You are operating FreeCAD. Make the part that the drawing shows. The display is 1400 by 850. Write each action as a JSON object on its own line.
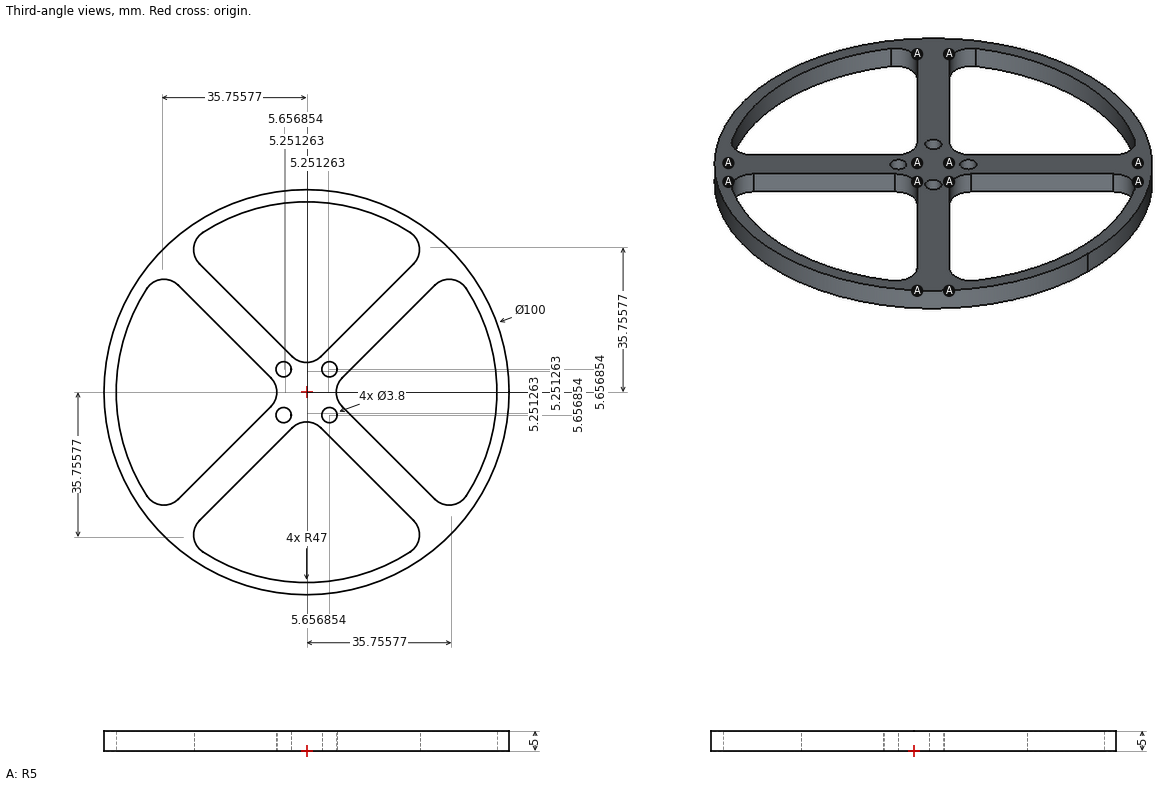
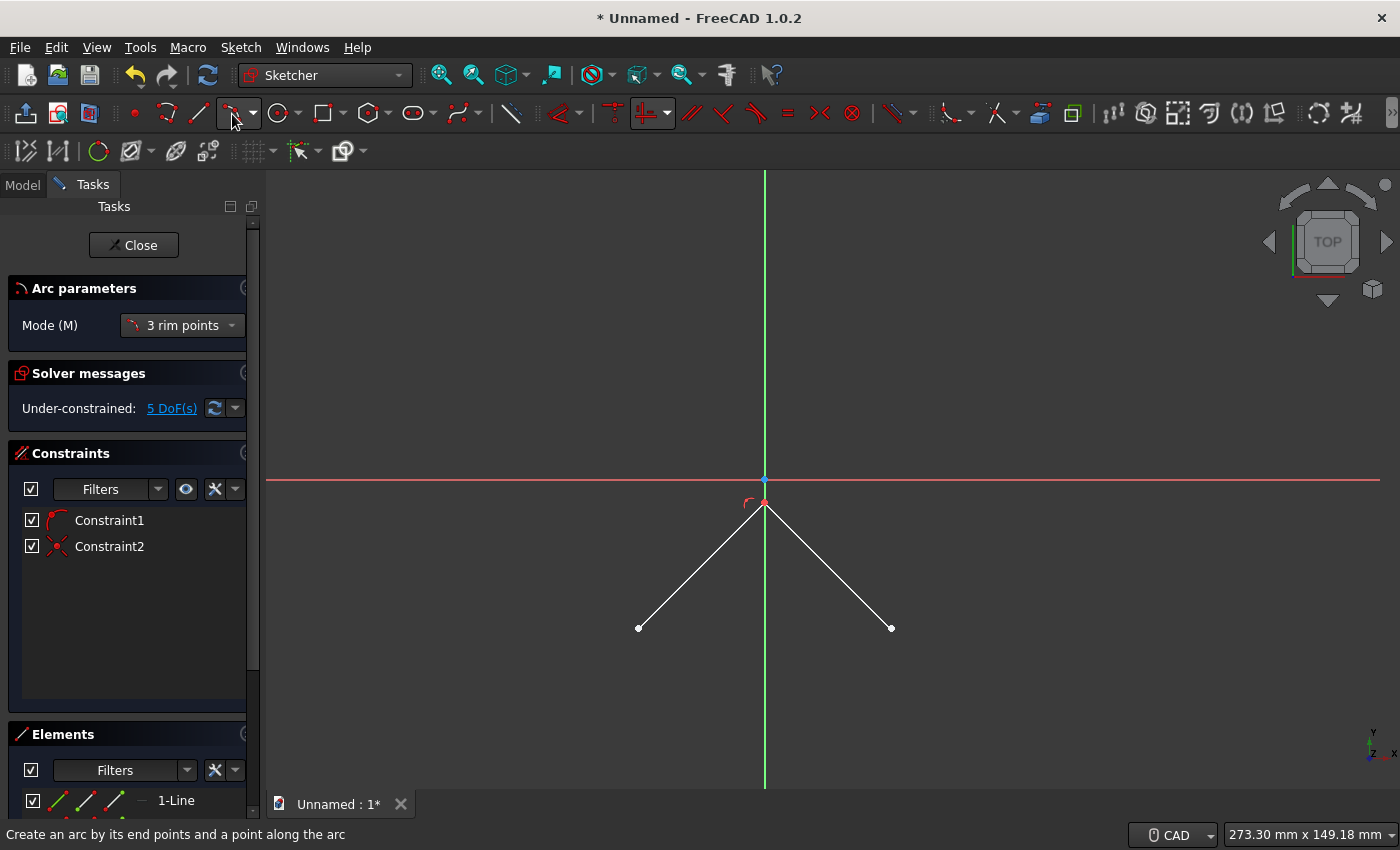
{"action": "left_click", "coordinate": [891, 629]}
{"action": "left_click", "coordinate": [638, 629]}
{"action": "left_click", "coordinate": [737, 673]}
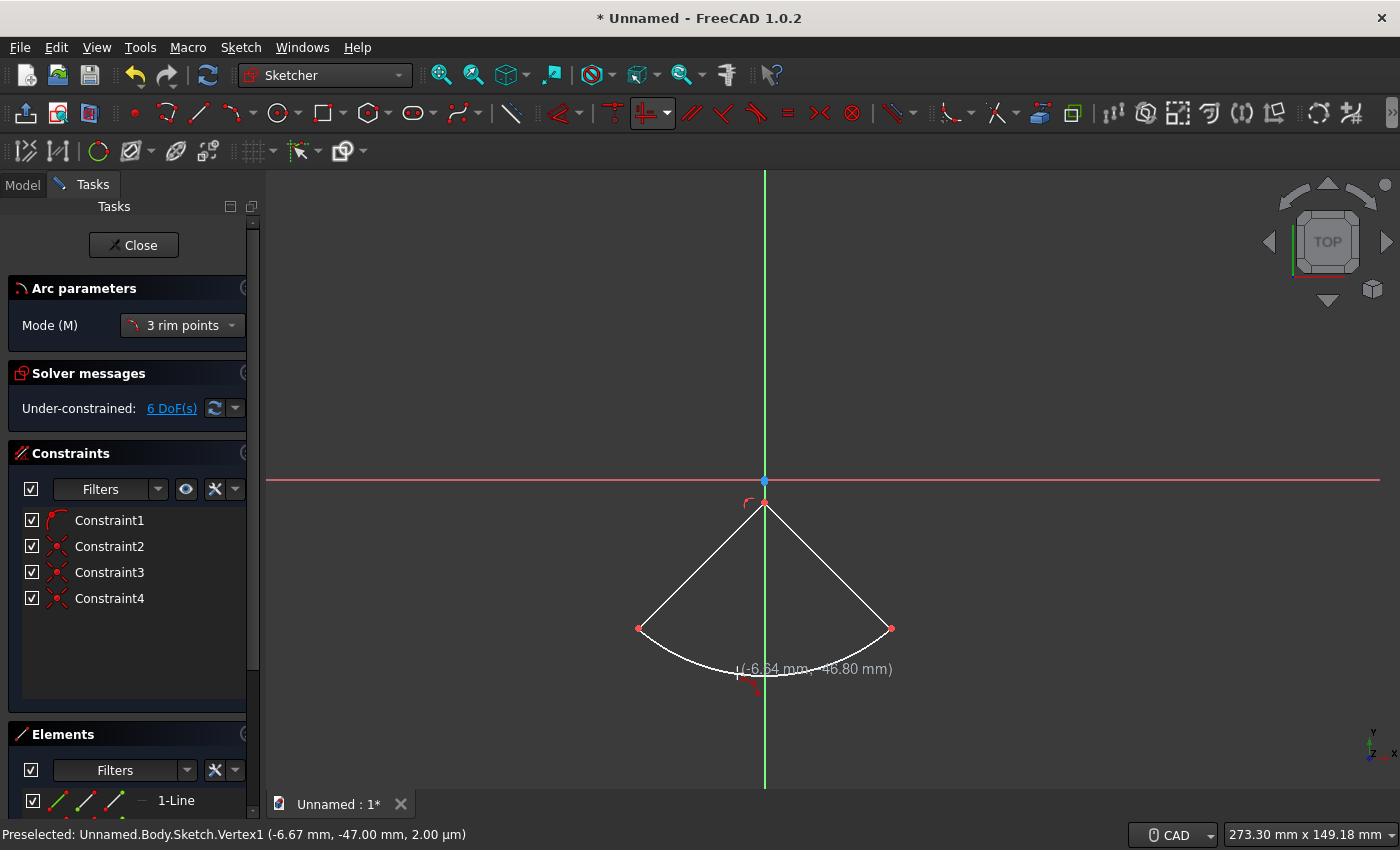
{"action": "left_click", "coordinate": [168, 114]}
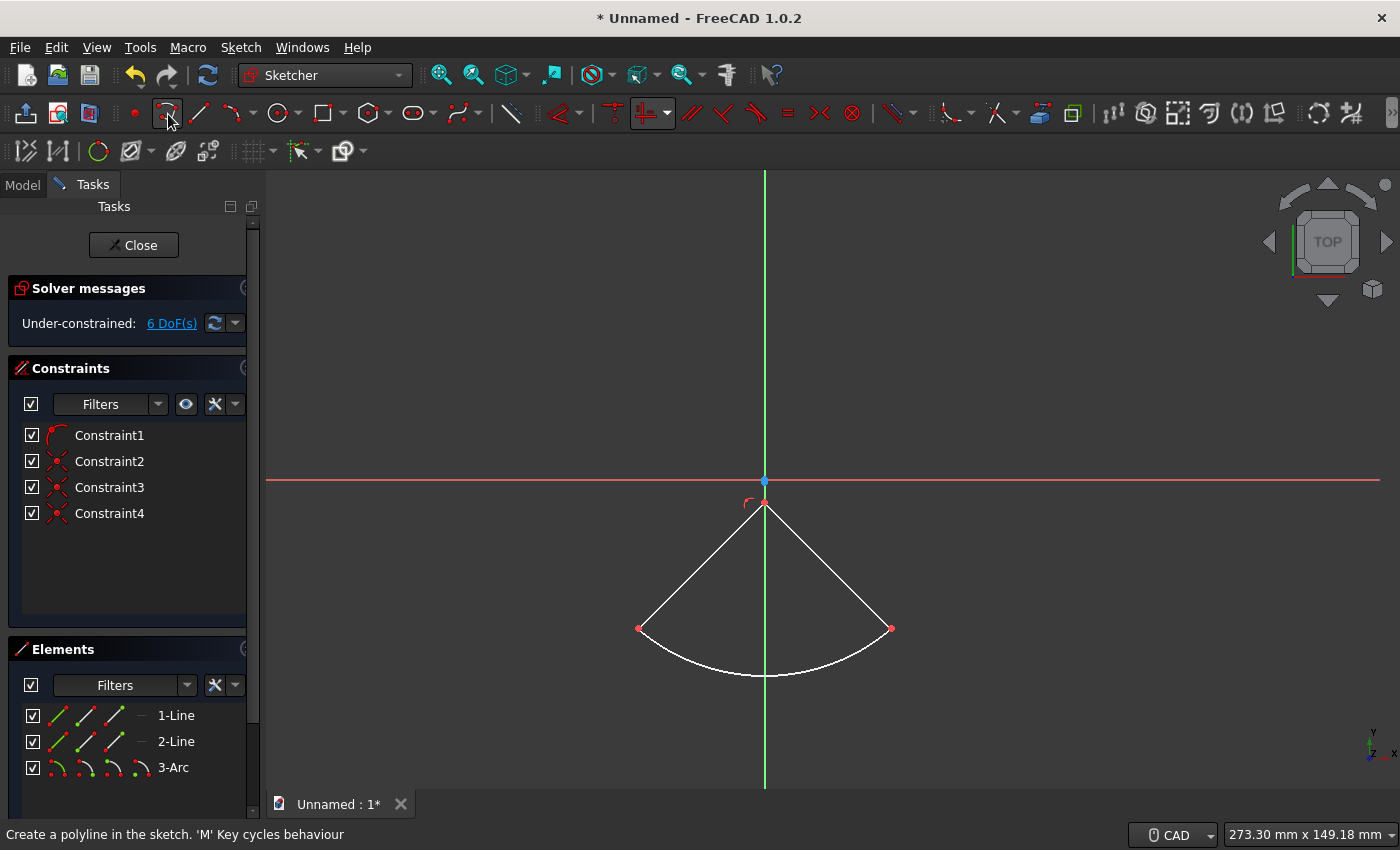
{"action": "left_click", "coordinate": [913, 606]}
{"action": "left_click", "coordinate": [786, 480]}
{"action": "left_click", "coordinate": [913, 353]}
{"action": "right_click", "coordinate": [913, 353]}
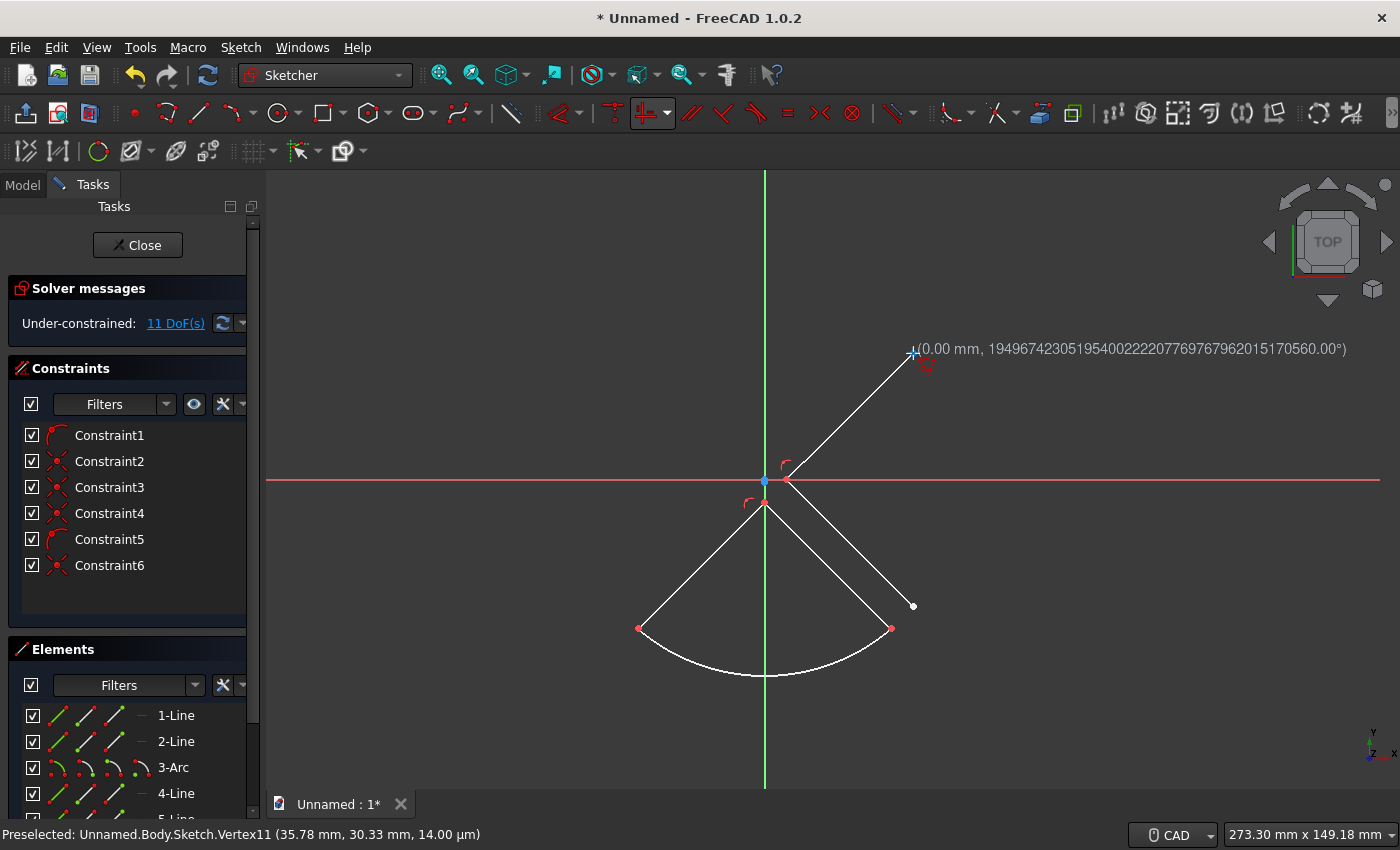
{"action": "left_click", "coordinate": [232, 114]}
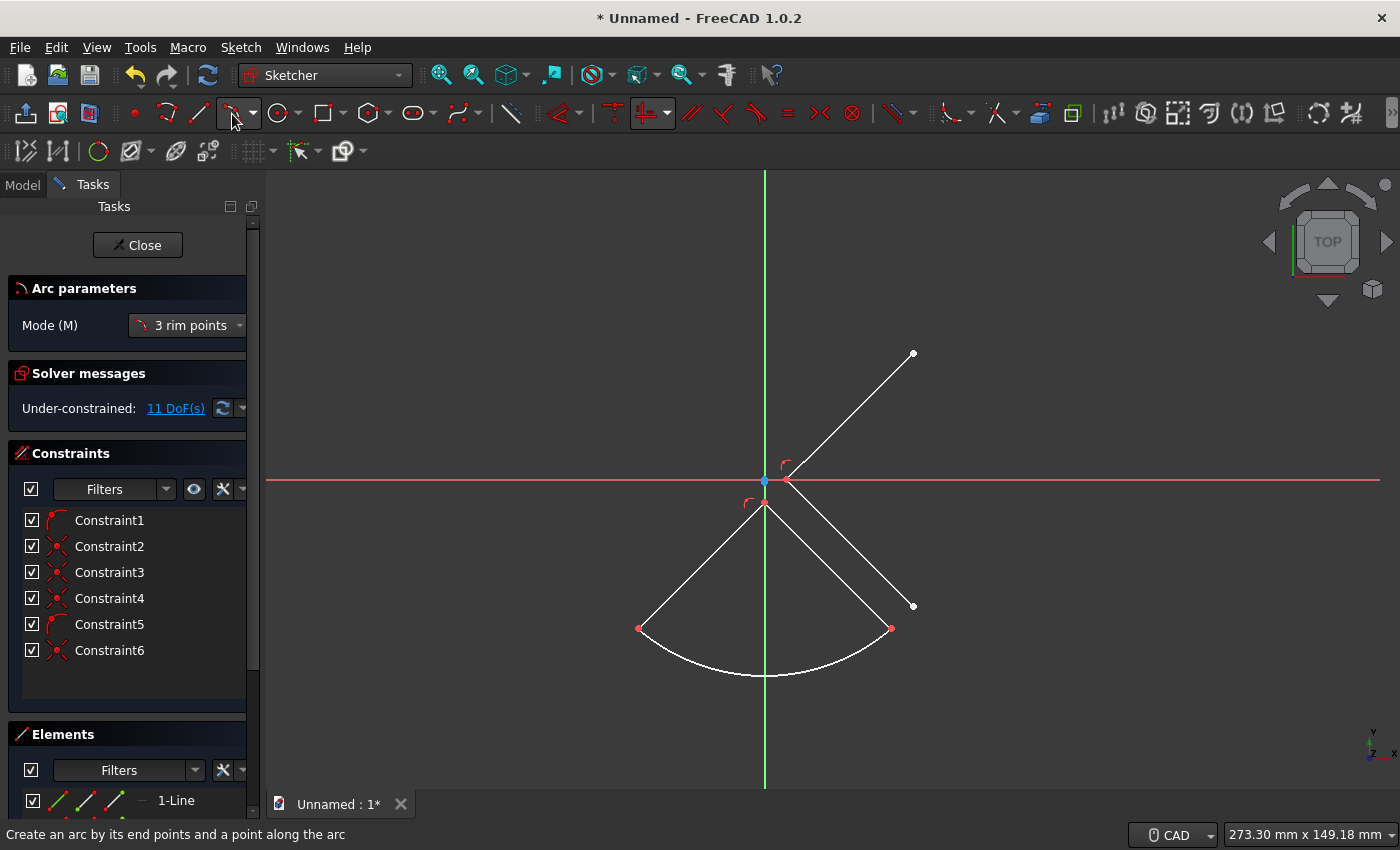
{"action": "left_click", "coordinate": [913, 354]}
{"action": "left_click", "coordinate": [913, 607]}
{"action": "left_click", "coordinate": [958, 507]}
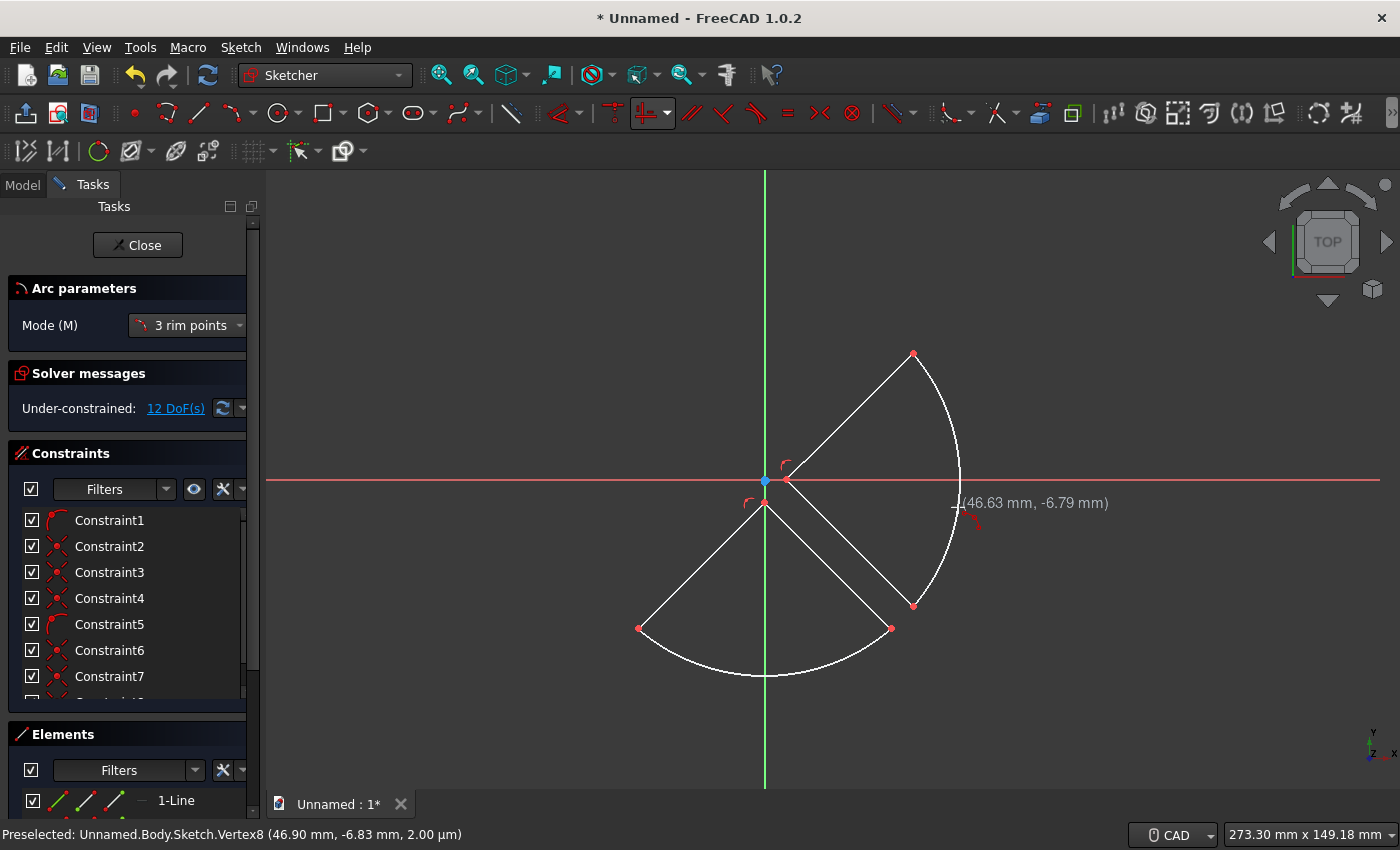
{"action": "left_click", "coordinate": [168, 114]}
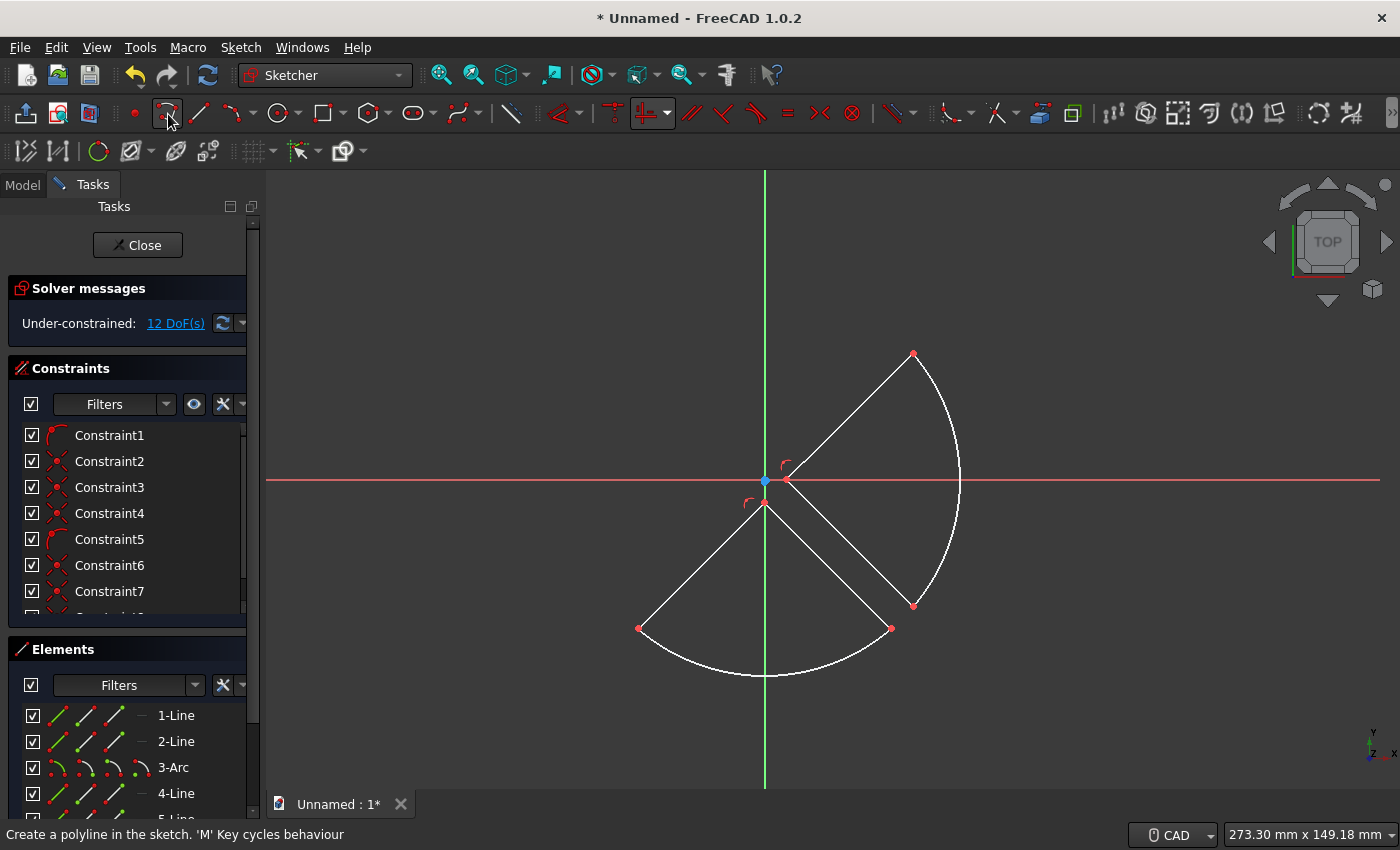
{"action": "left_click", "coordinate": [616, 353]}
{"action": "left_click", "coordinate": [743, 480]}
{"action": "left_click", "coordinate": [616, 606]}
{"action": "right_click", "coordinate": [616, 606]}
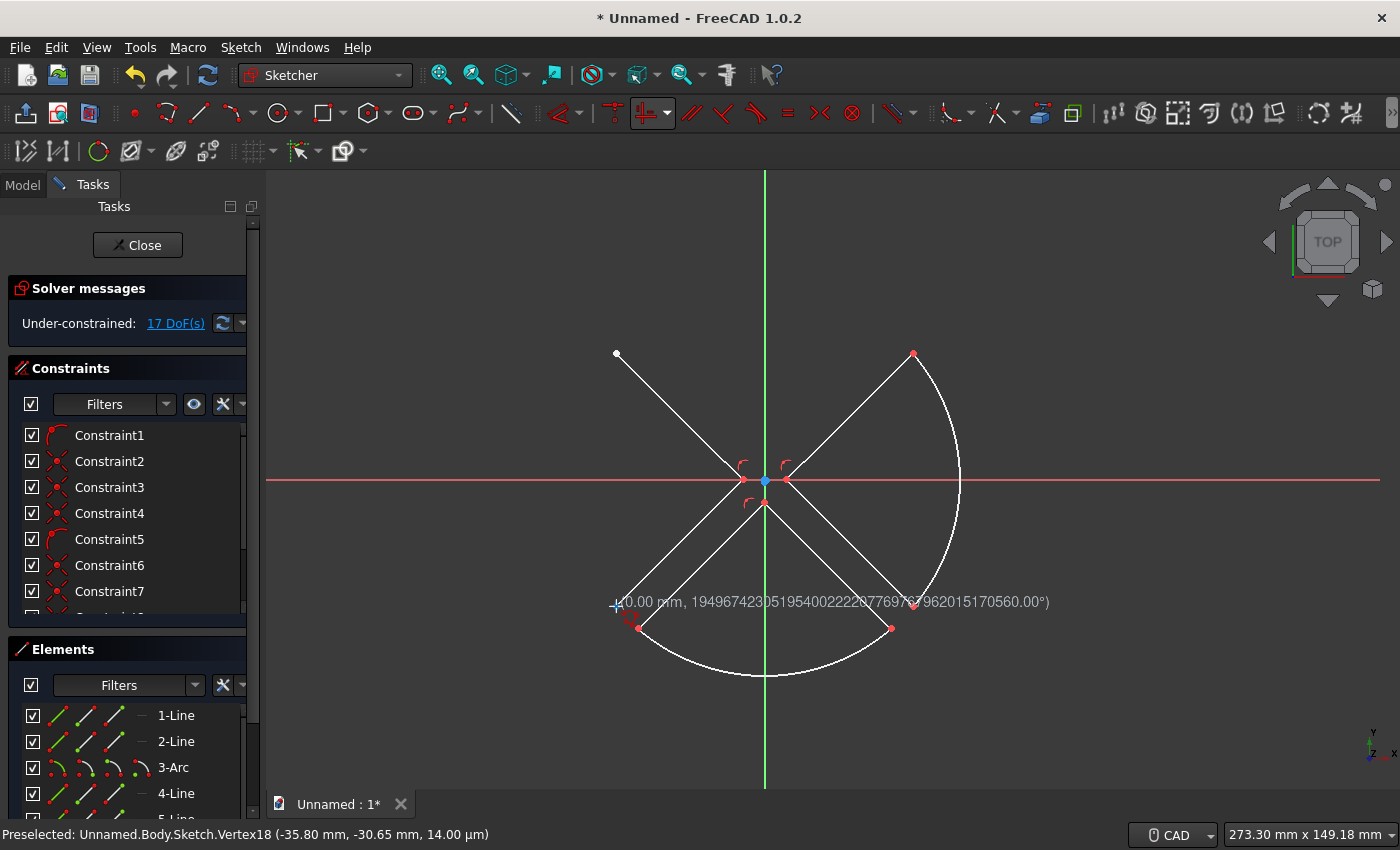
{"action": "left_click", "coordinate": [232, 114]}